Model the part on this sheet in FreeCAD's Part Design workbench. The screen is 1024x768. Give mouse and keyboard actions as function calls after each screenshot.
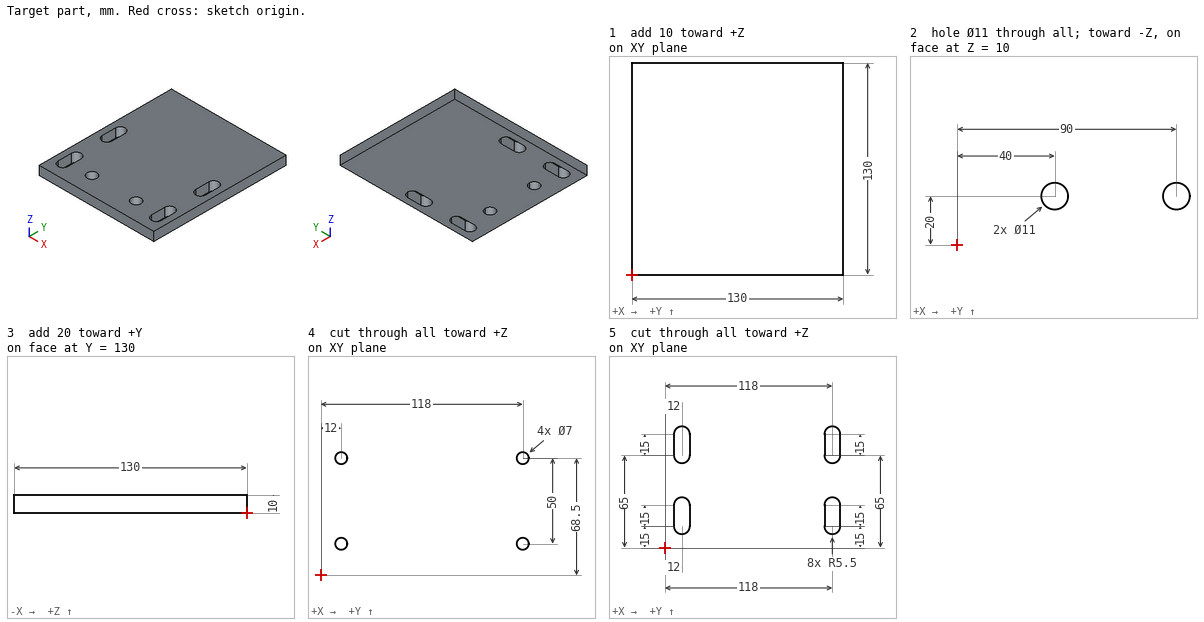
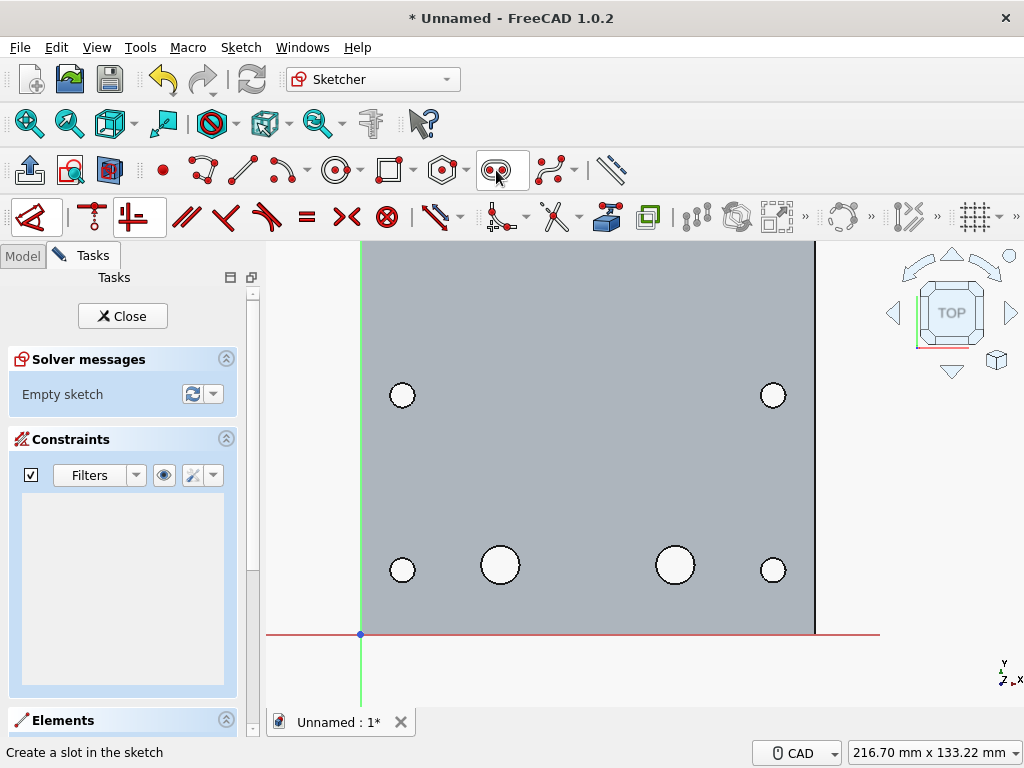
click(773, 583)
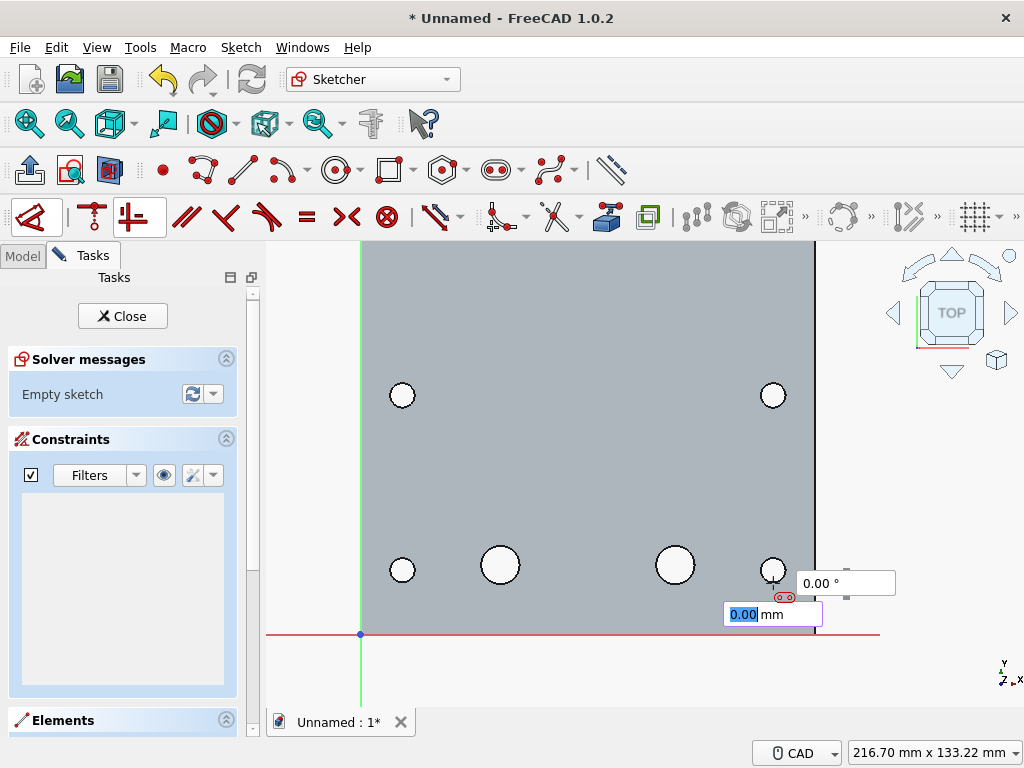
click(773, 530)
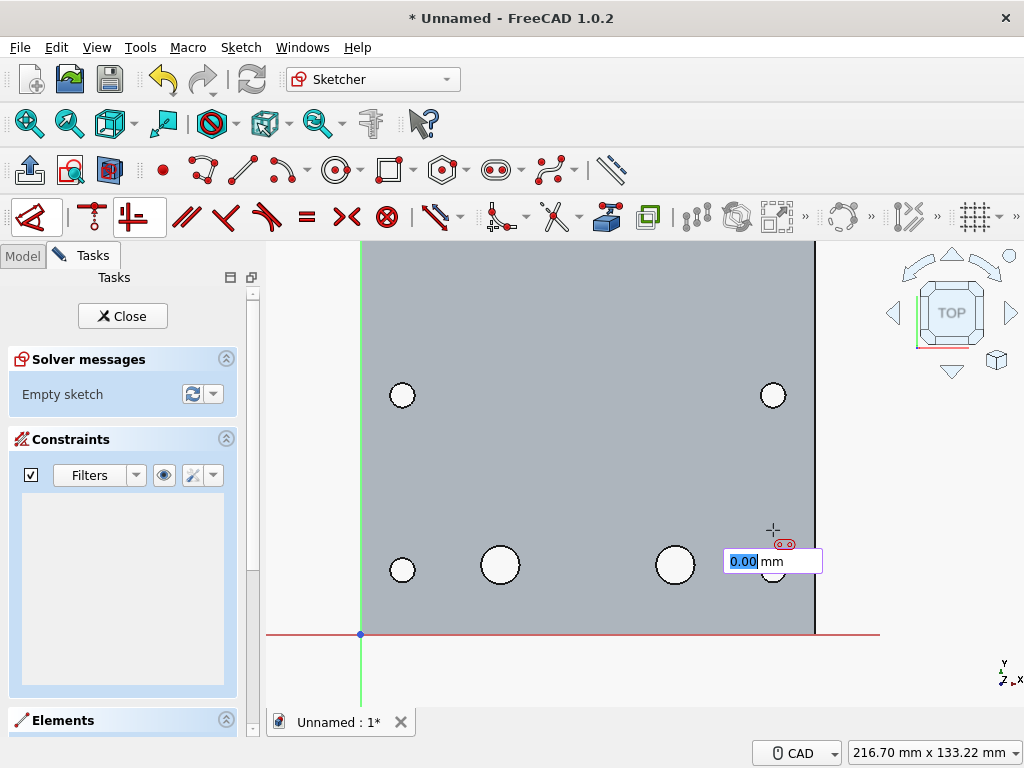
click(792, 556)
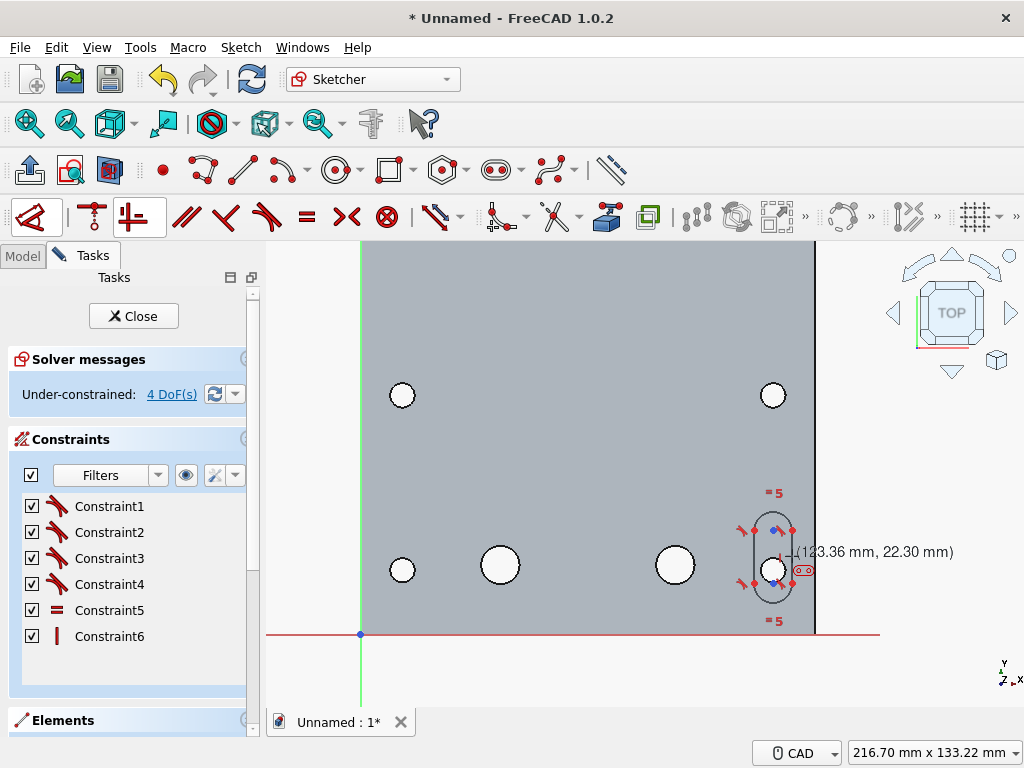
click(773, 408)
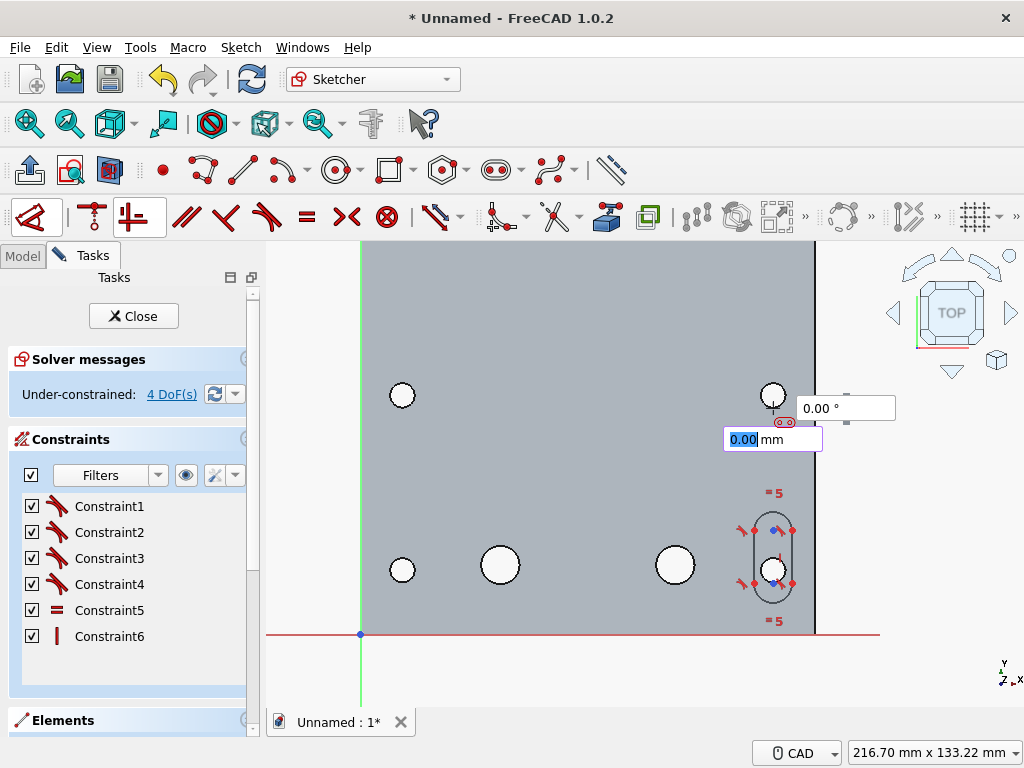
click(773, 355)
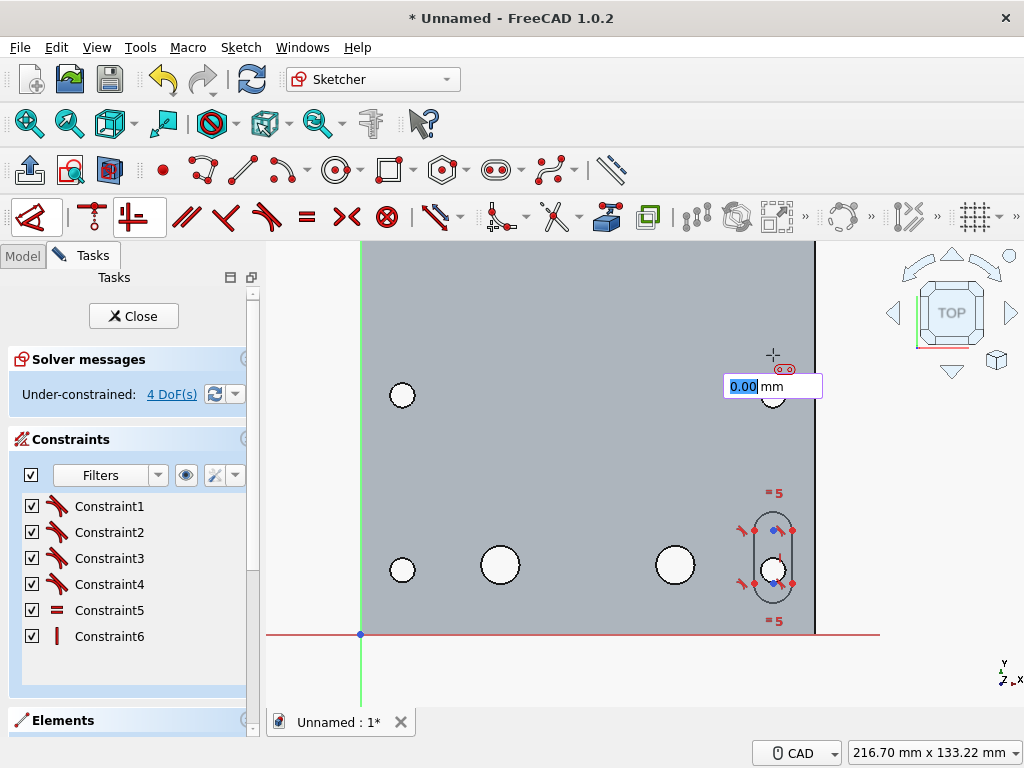
click(792, 381)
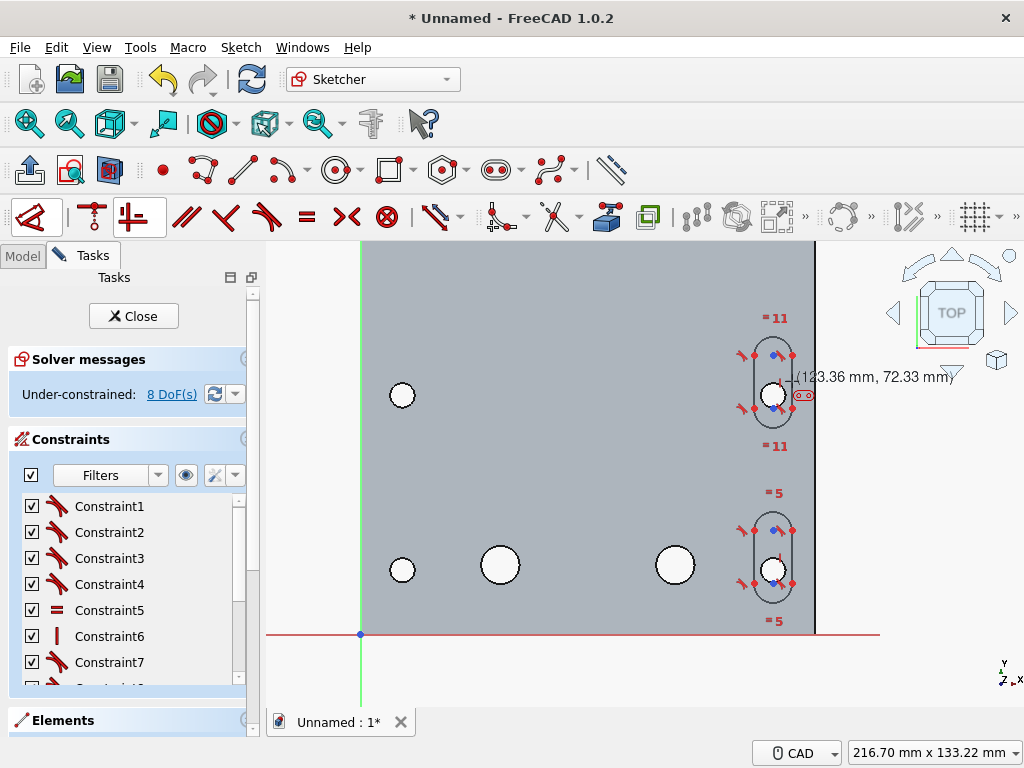
click(402, 408)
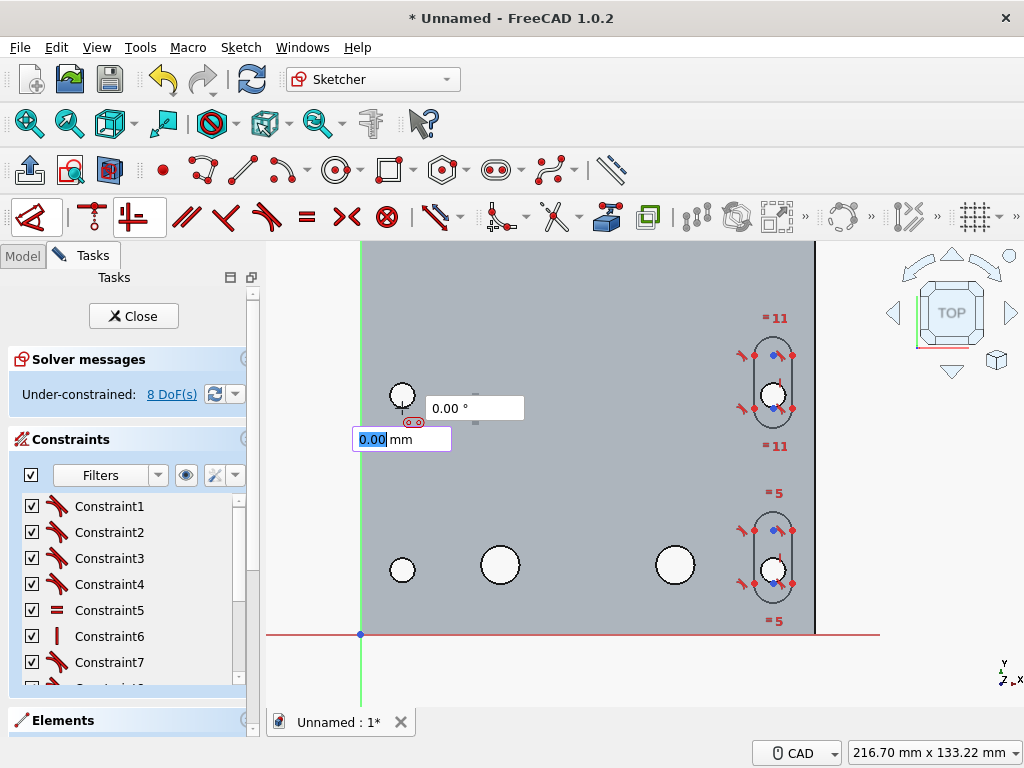
click(402, 355)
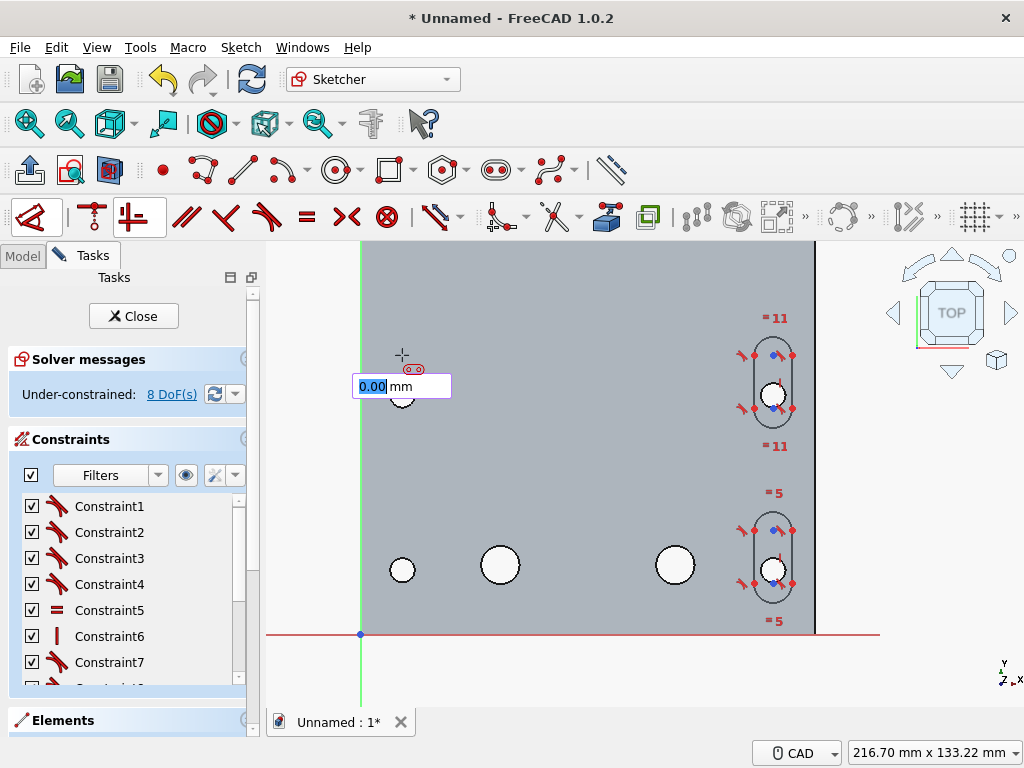
click(422, 381)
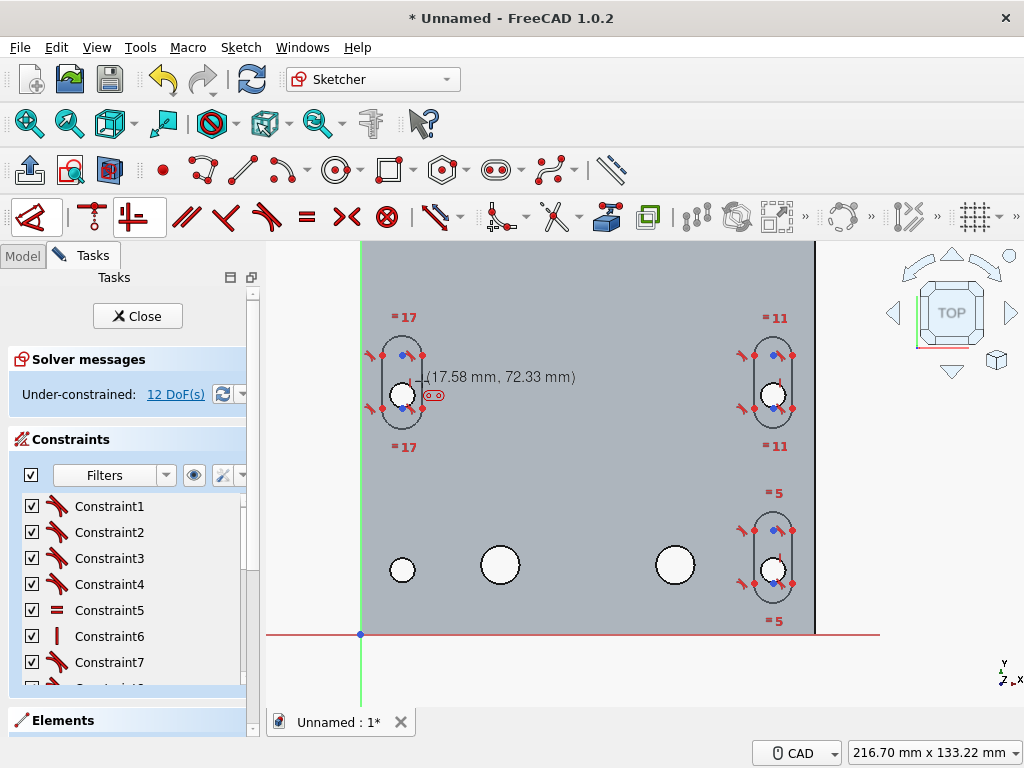
click(402, 583)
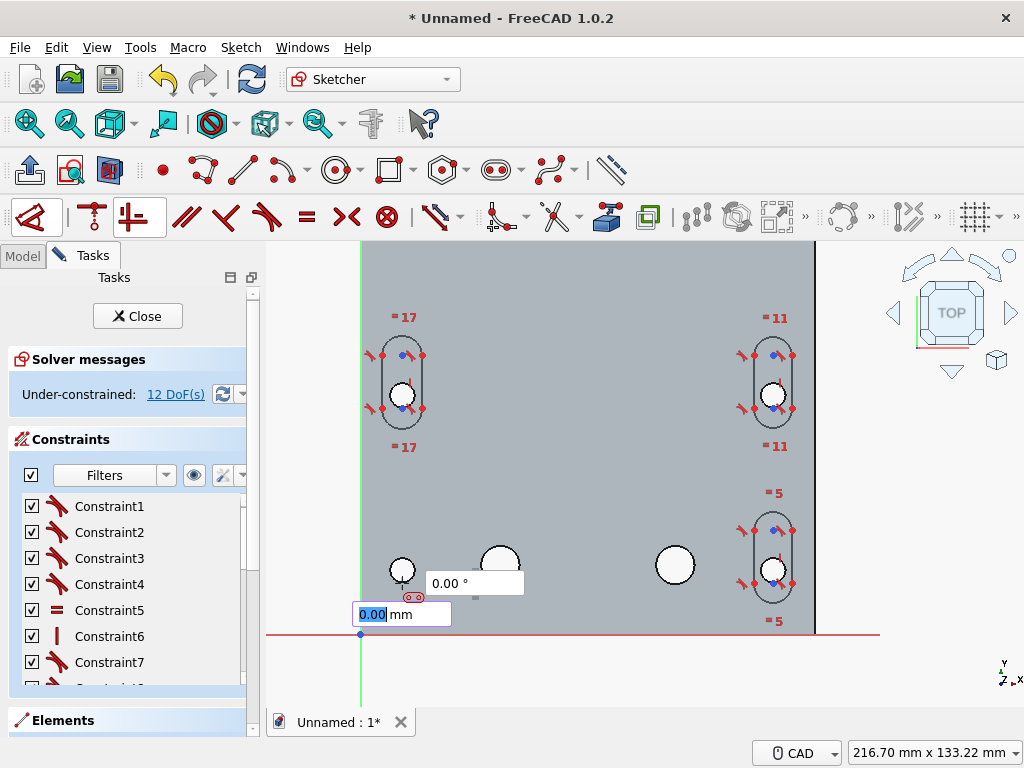
click(402, 530)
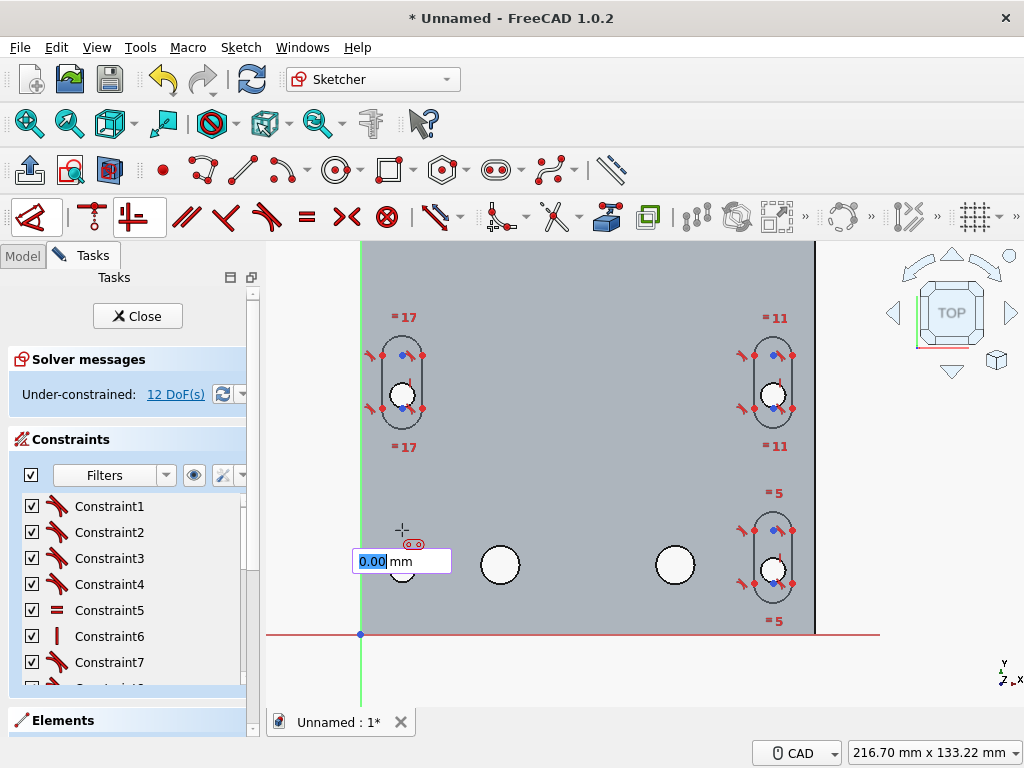
click(422, 556)
key(Escape)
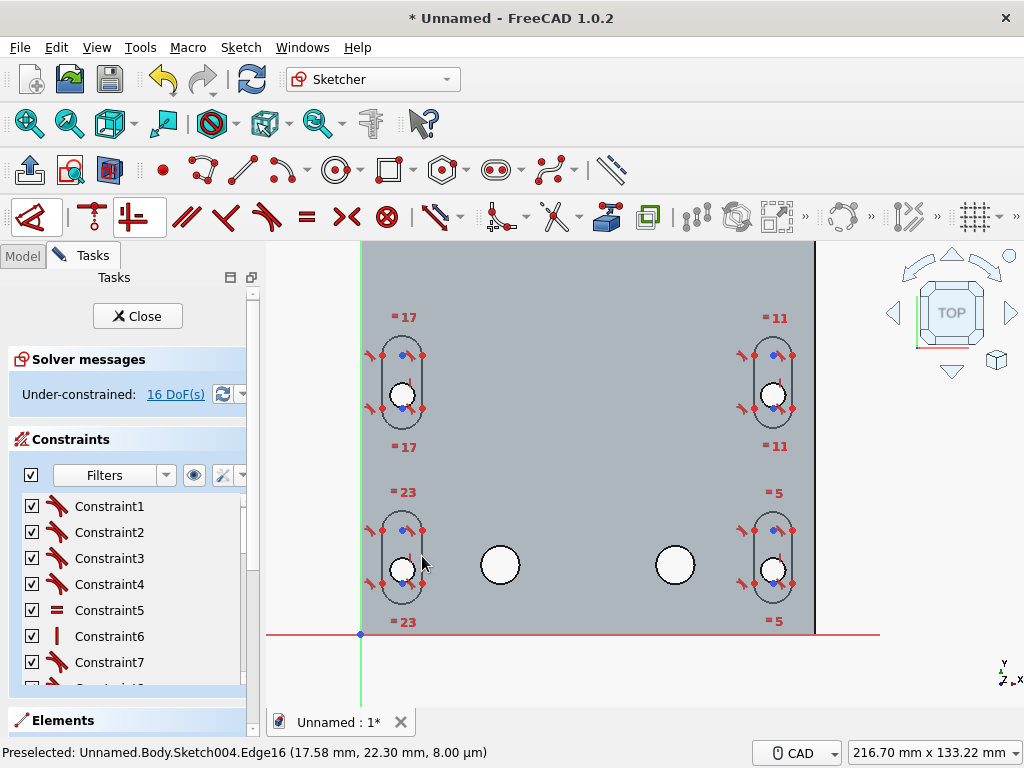
click(762, 599)